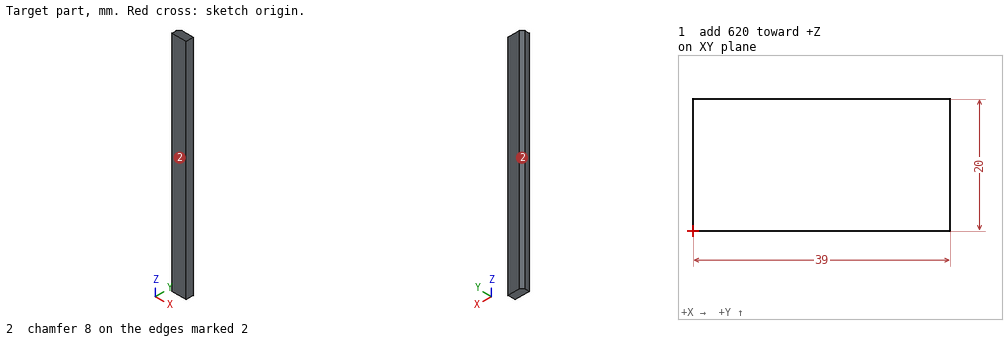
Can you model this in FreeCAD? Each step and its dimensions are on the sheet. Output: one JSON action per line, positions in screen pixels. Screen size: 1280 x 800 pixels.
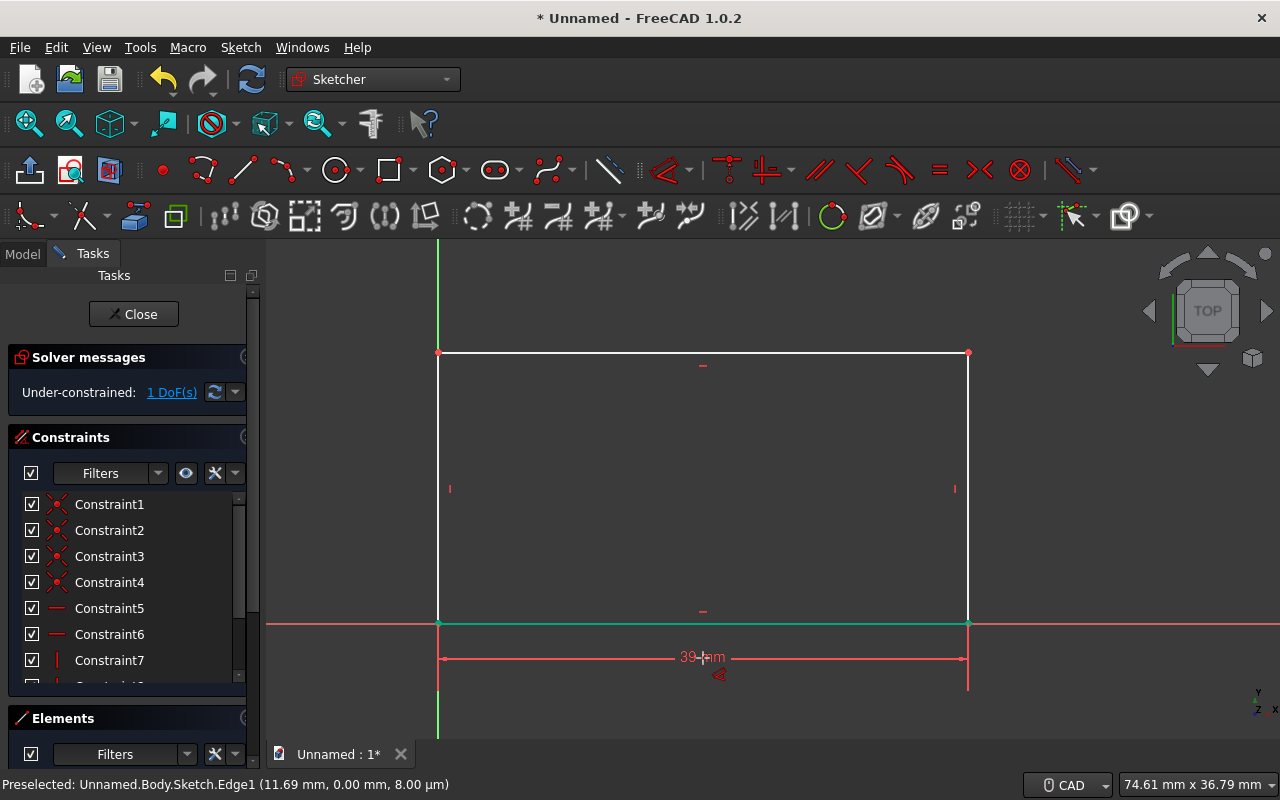
{"action": "left_click", "coordinate": [968, 542]}
{"action": "left_click", "coordinate": [1002, 488]}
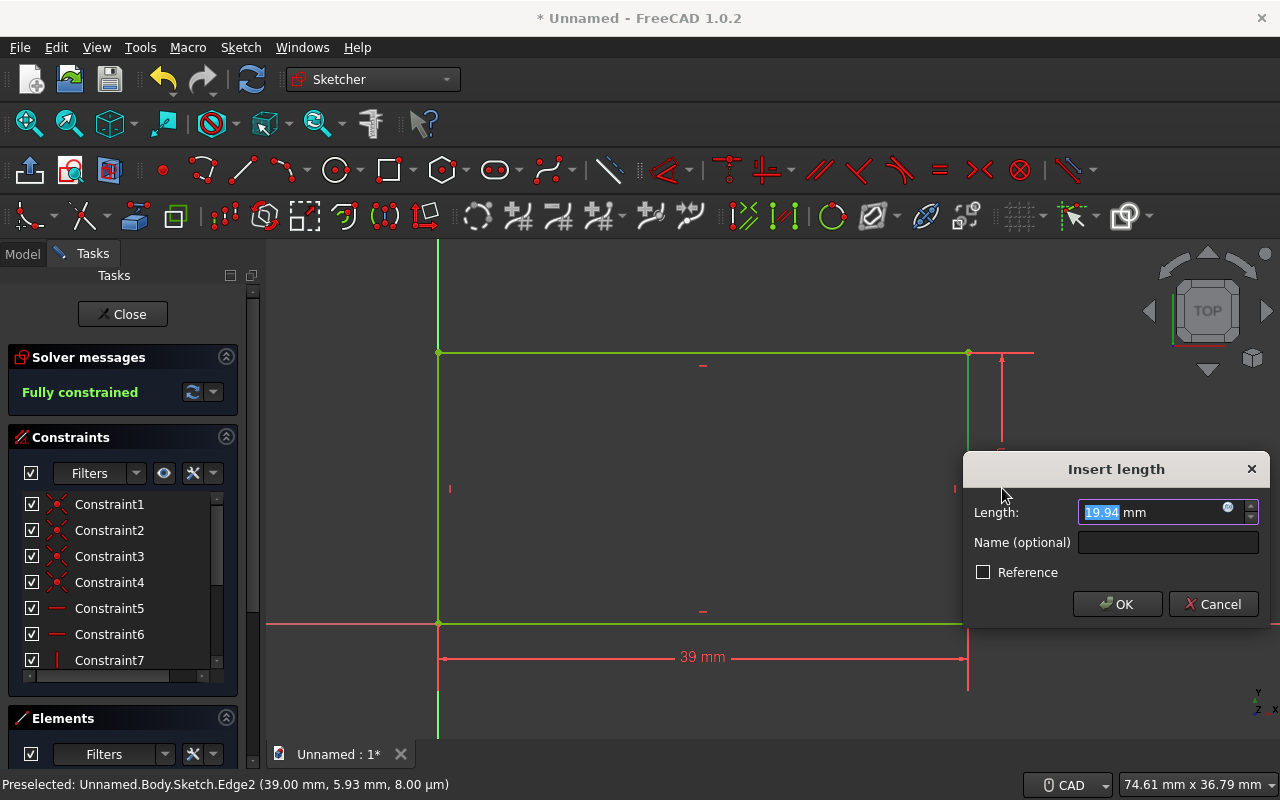
{"action": "type", "text": "20"}
{"action": "key", "text": "Return"}
{"action": "key", "text": "Escape"}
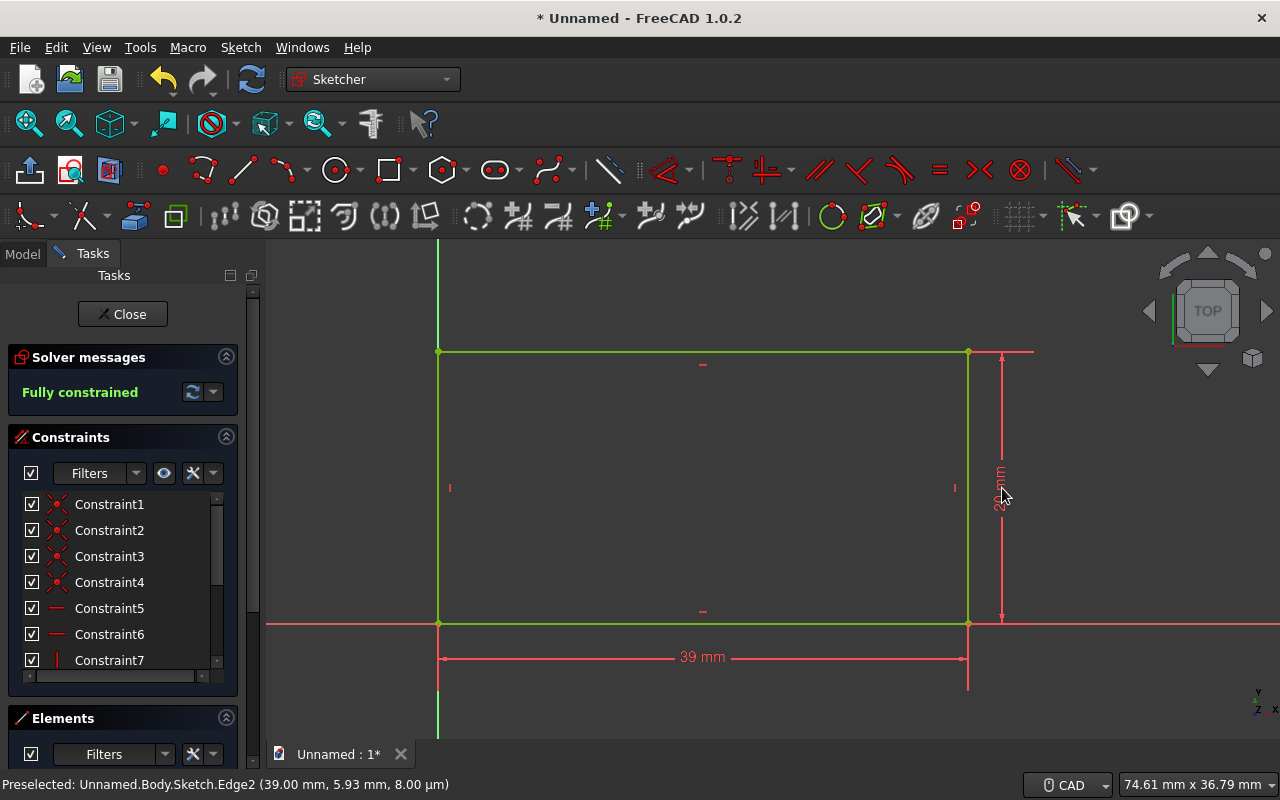
{"action": "left_click", "coordinate": [123, 314]}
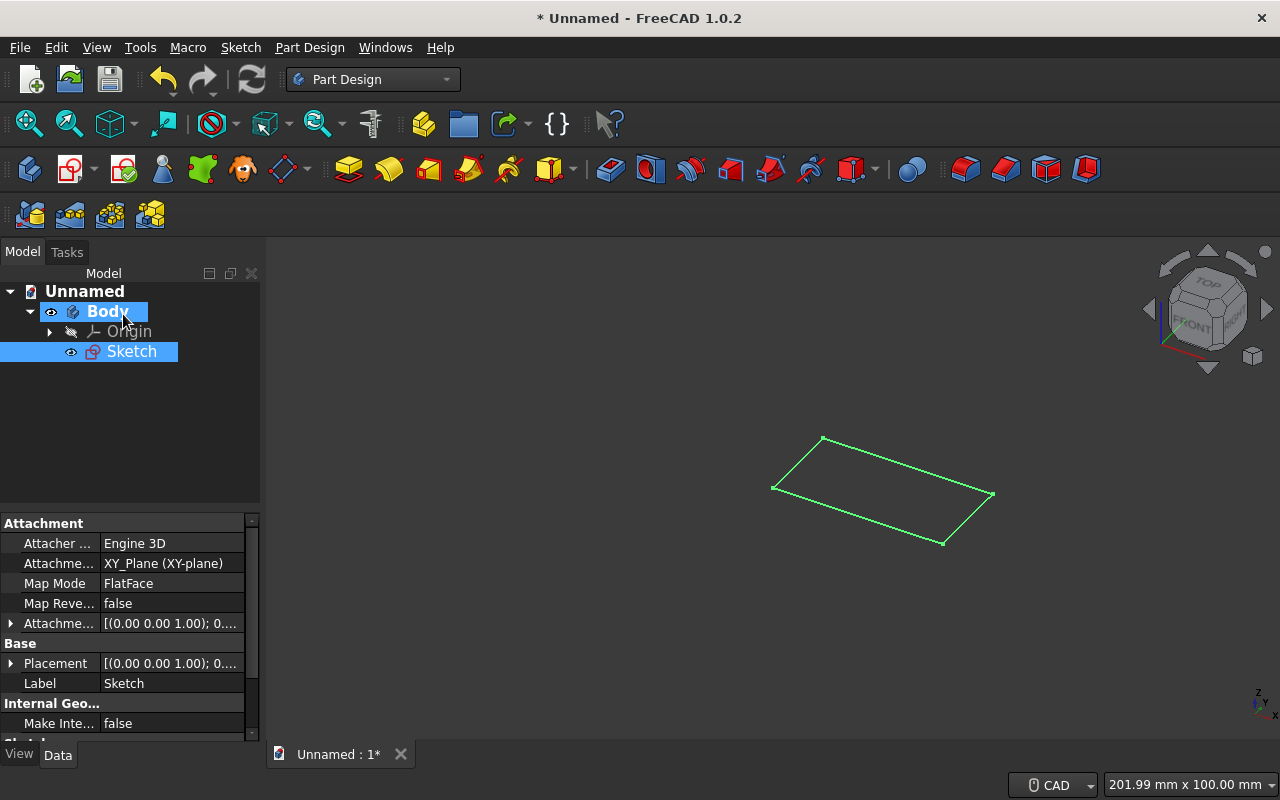
{"action": "left_click", "coordinate": [350, 170]}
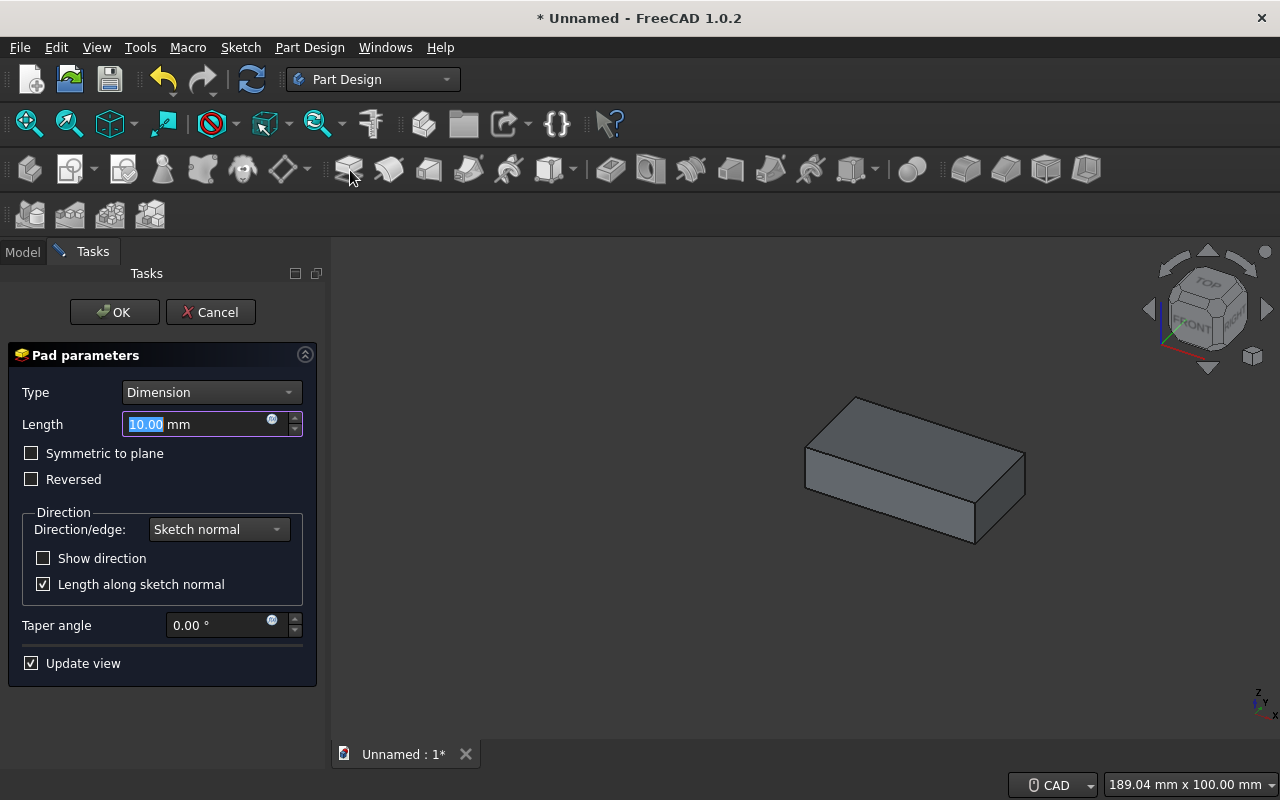
{"action": "type", "text": "620"}
{"action": "key", "text": "Tab"}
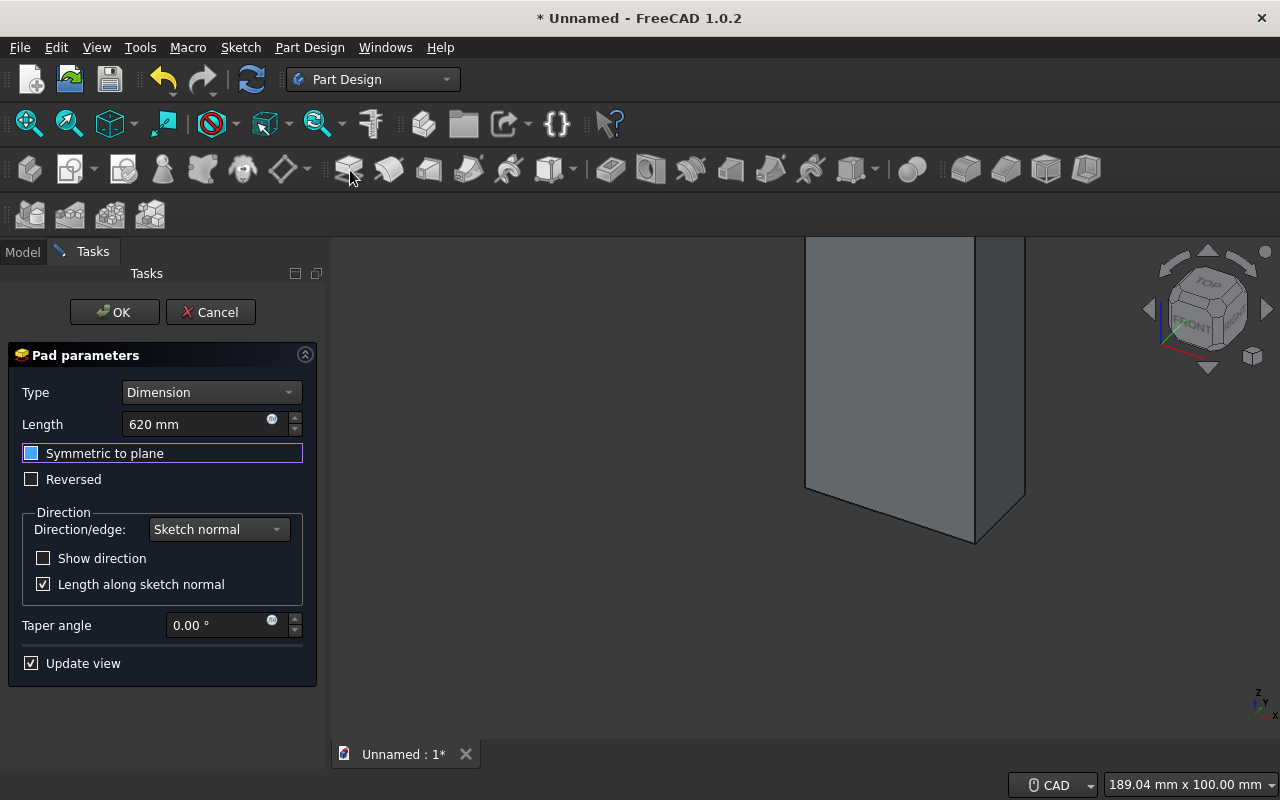
{"action": "left_click", "coordinate": [115, 312]}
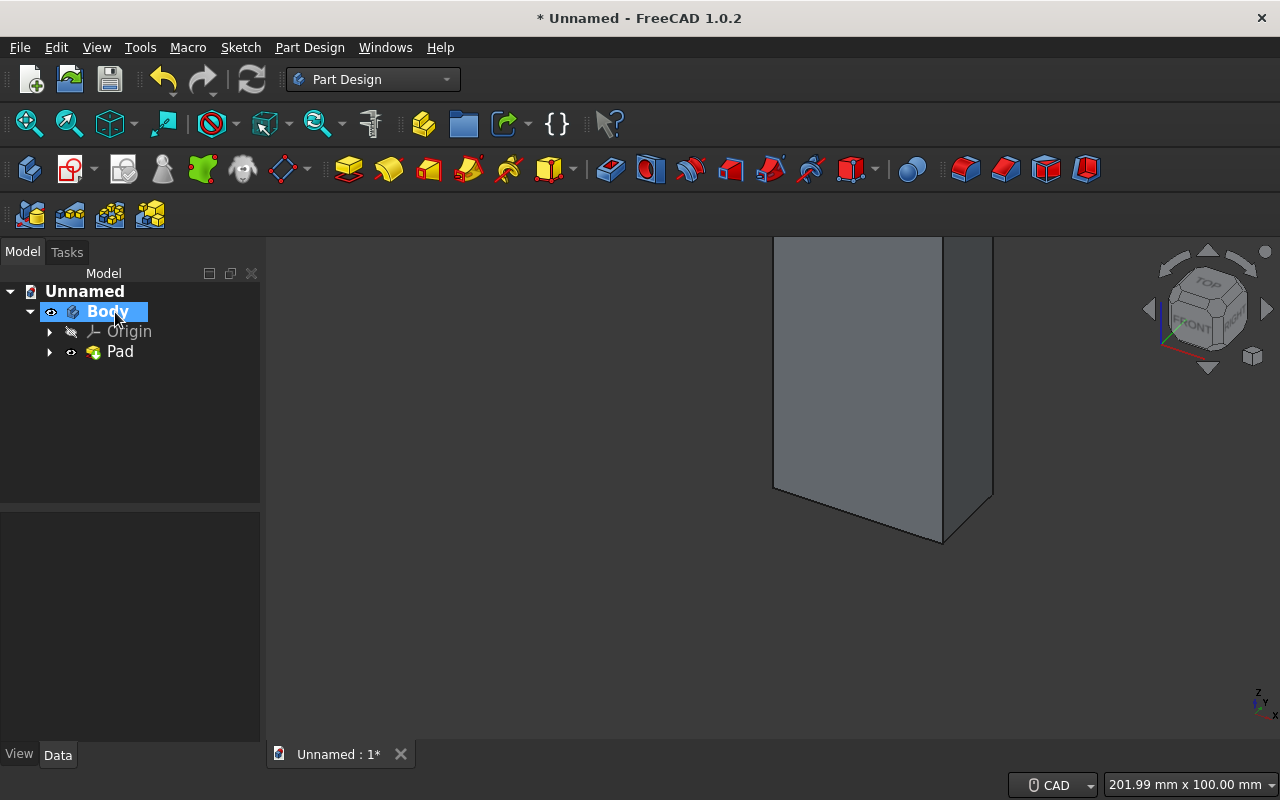
{"action": "key", "text": "v f"}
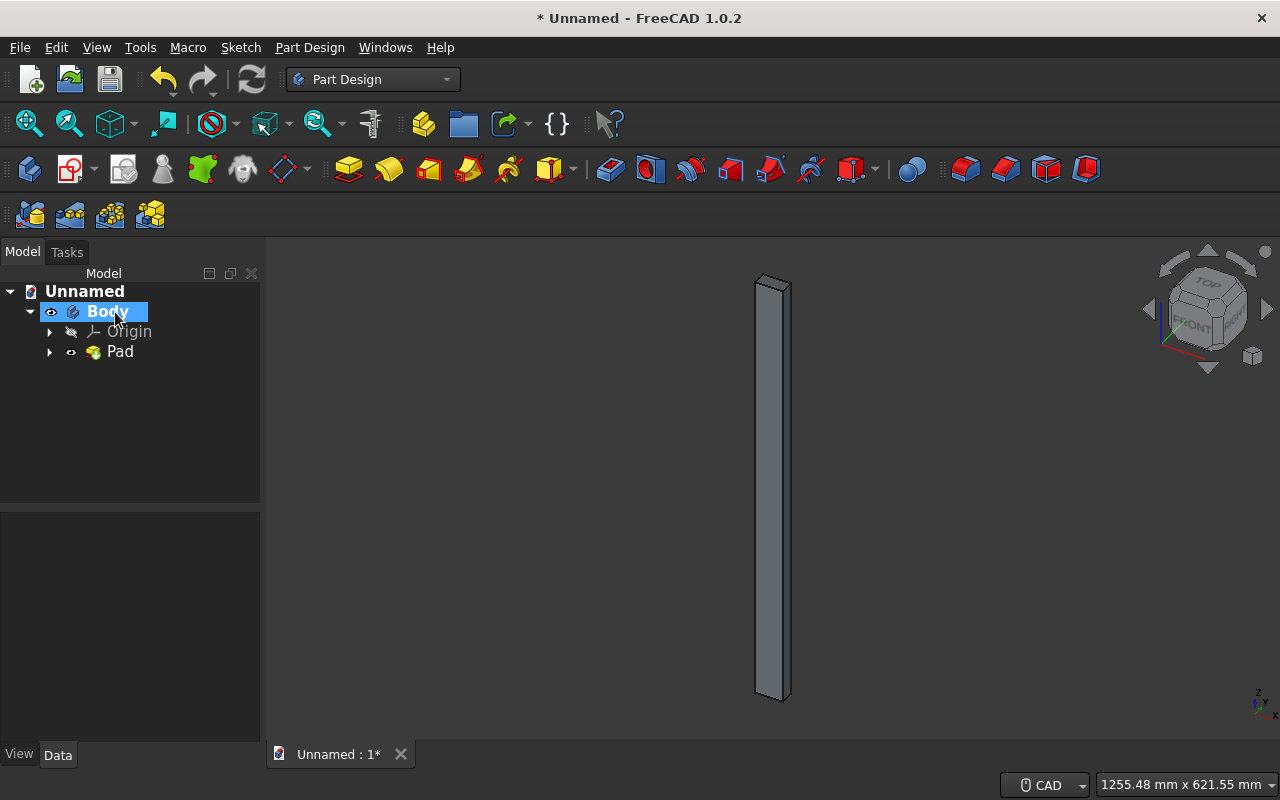
{"action": "key", "text": "0"}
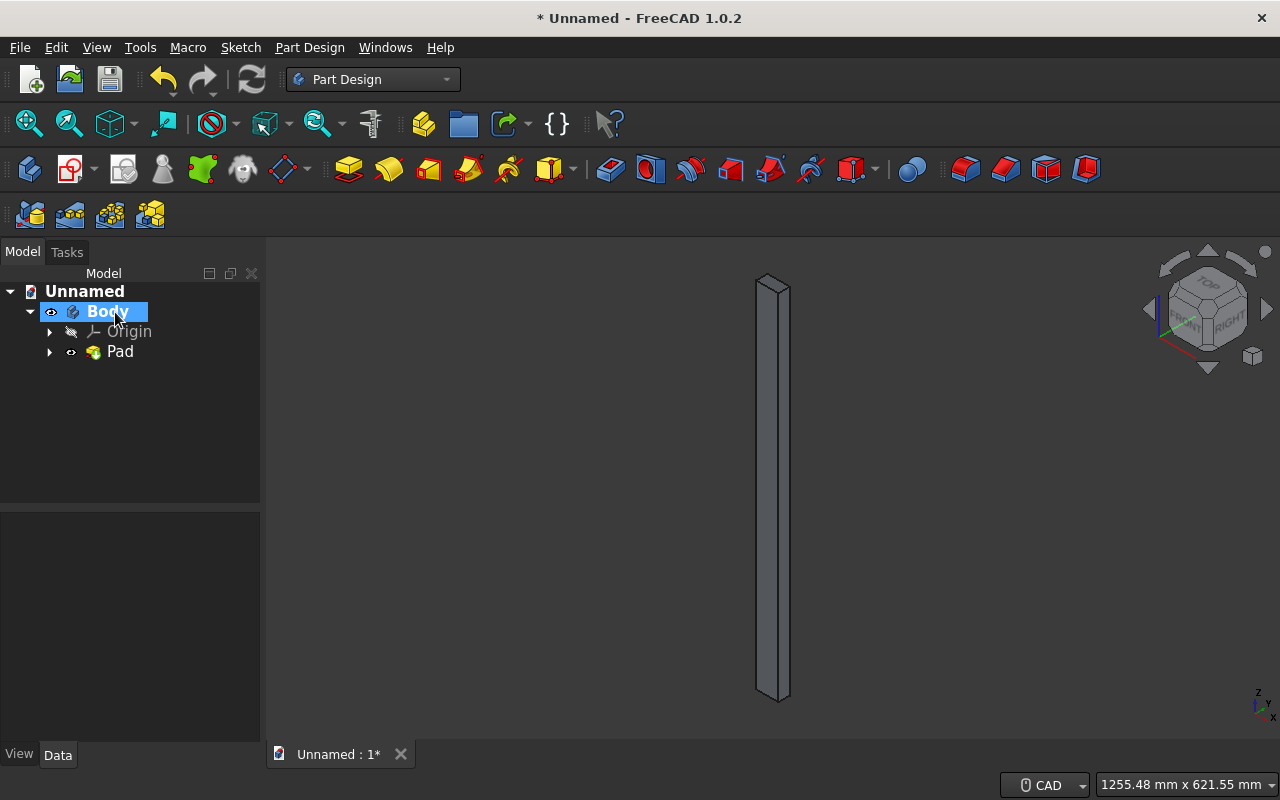
{"action": "key", "text": "2"}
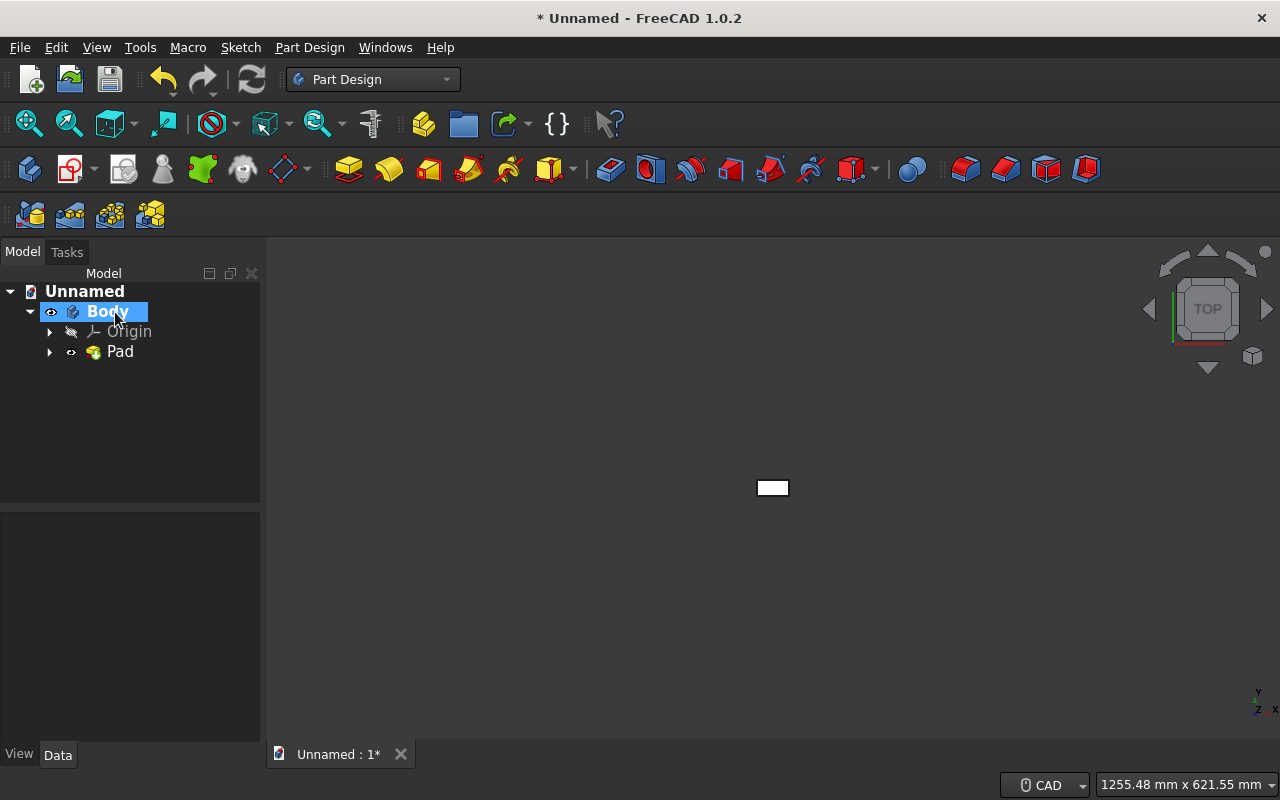
{"action": "key", "text": "v f"}